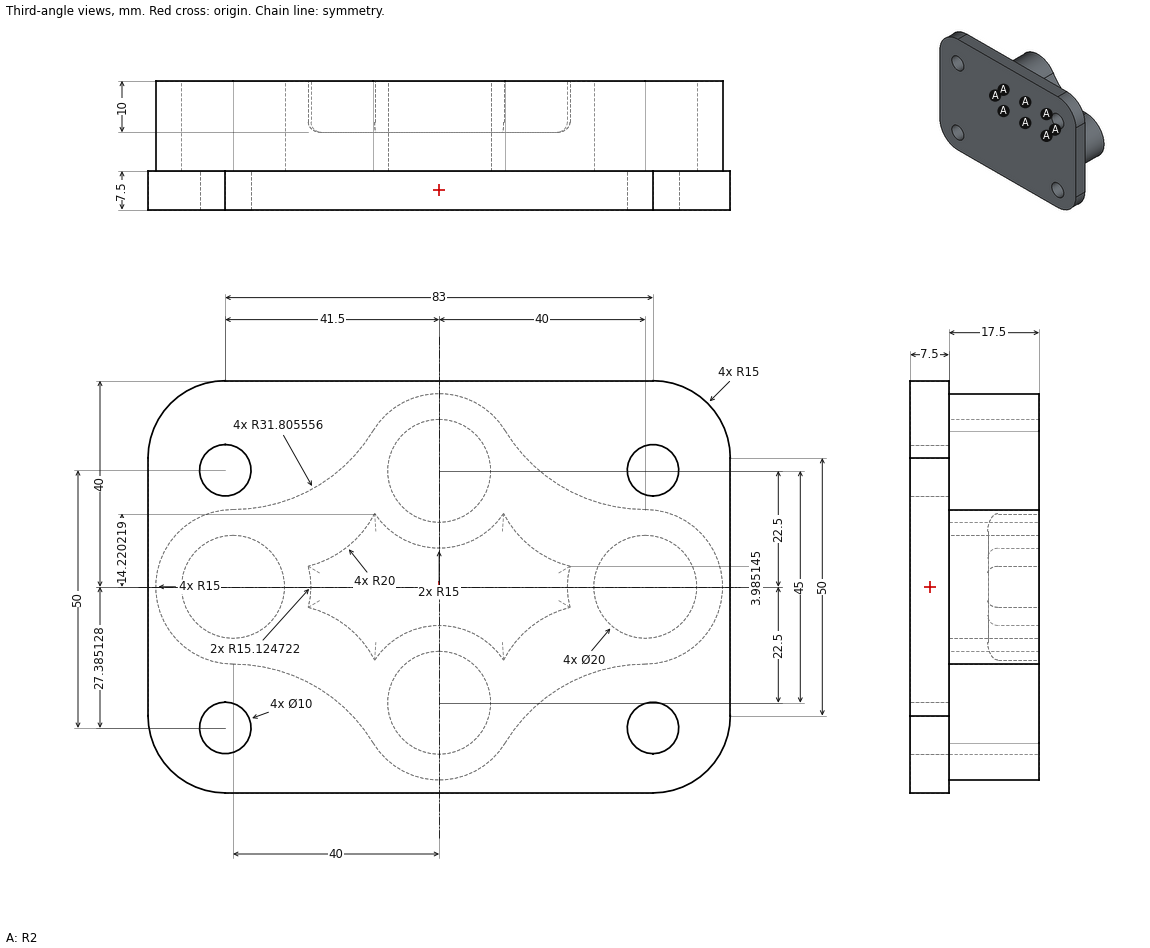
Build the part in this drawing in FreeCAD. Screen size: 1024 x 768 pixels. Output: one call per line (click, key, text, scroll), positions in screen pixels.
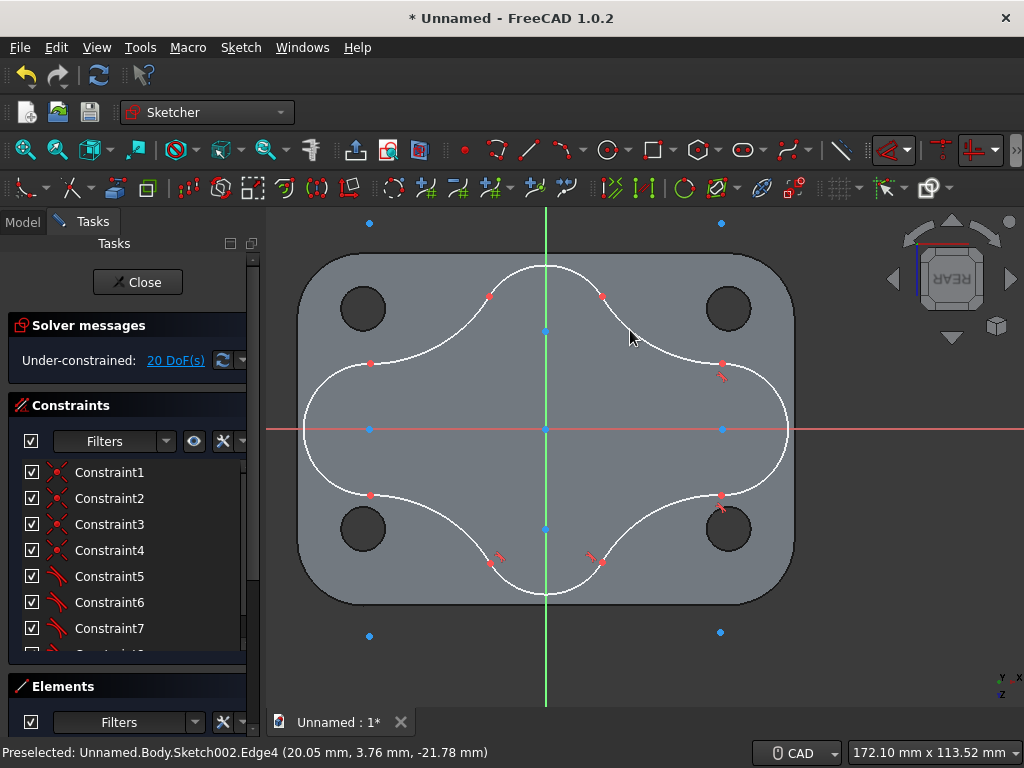
click(630, 330)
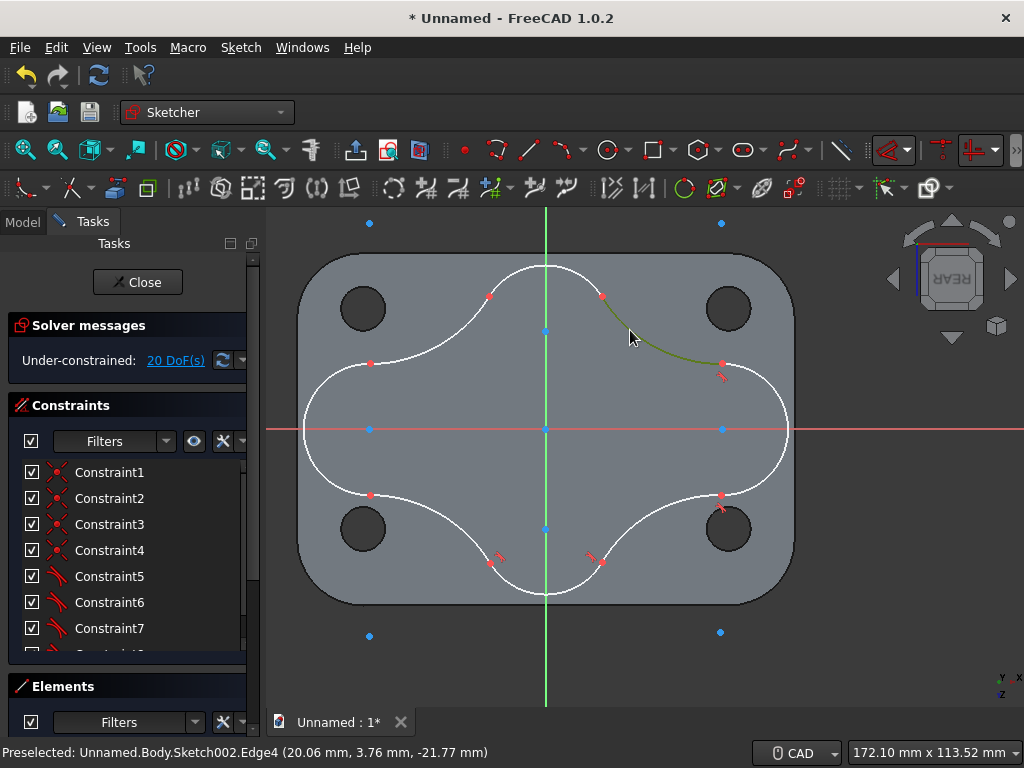
click(572, 271)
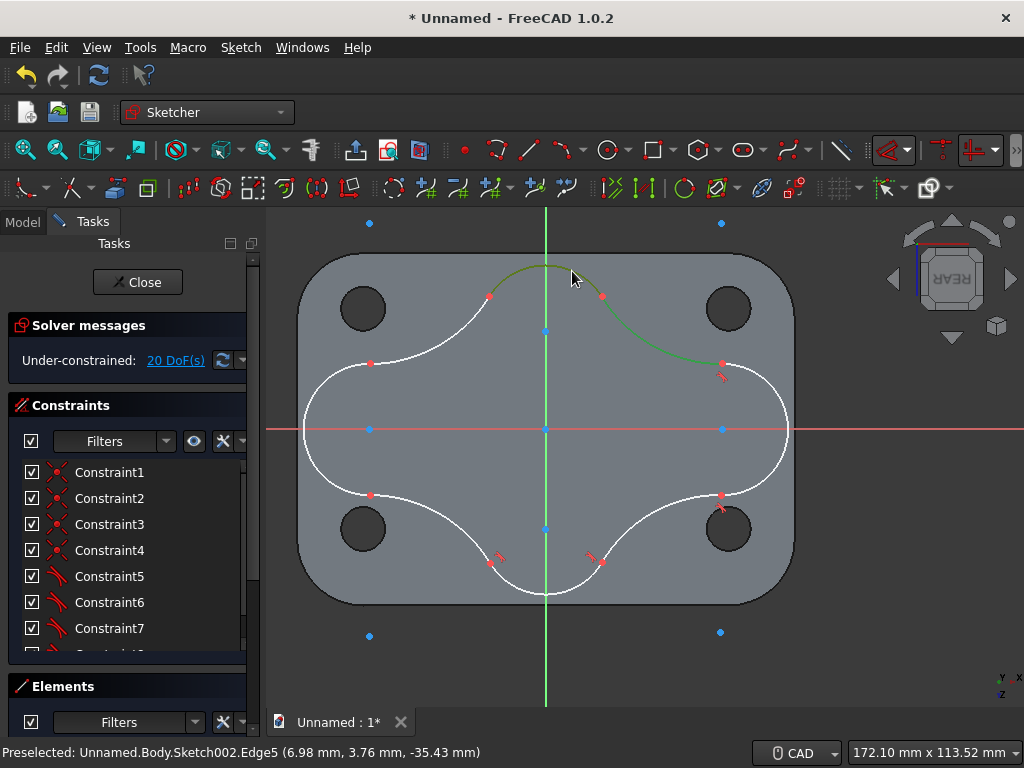
key(t)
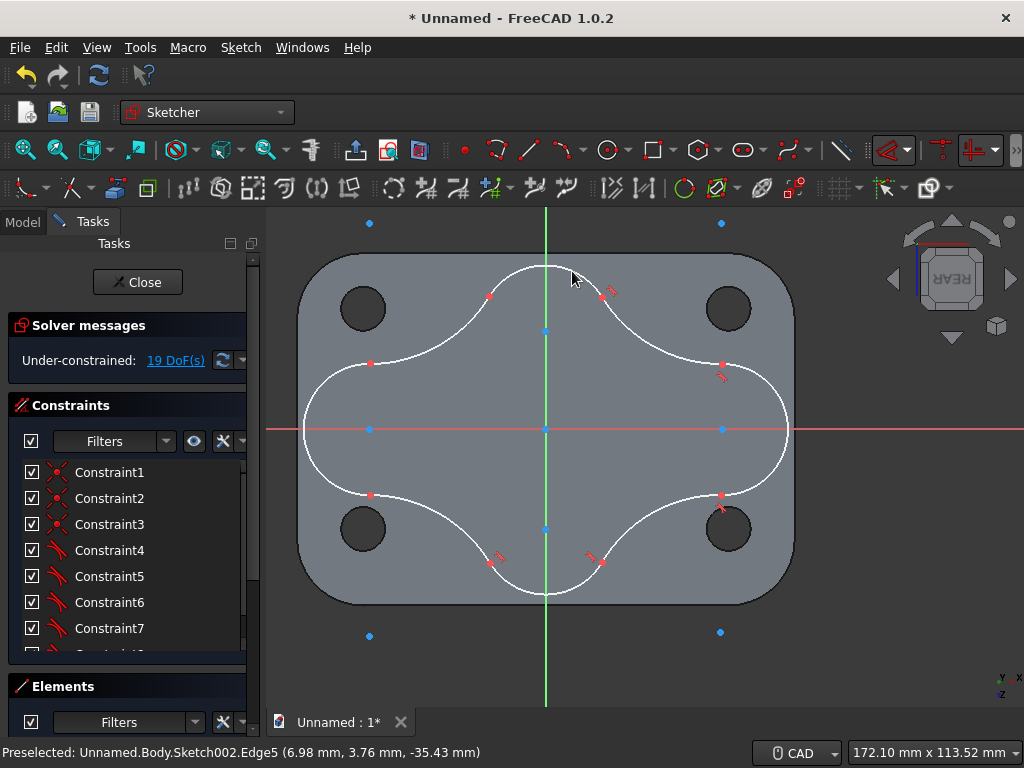
click(572, 271)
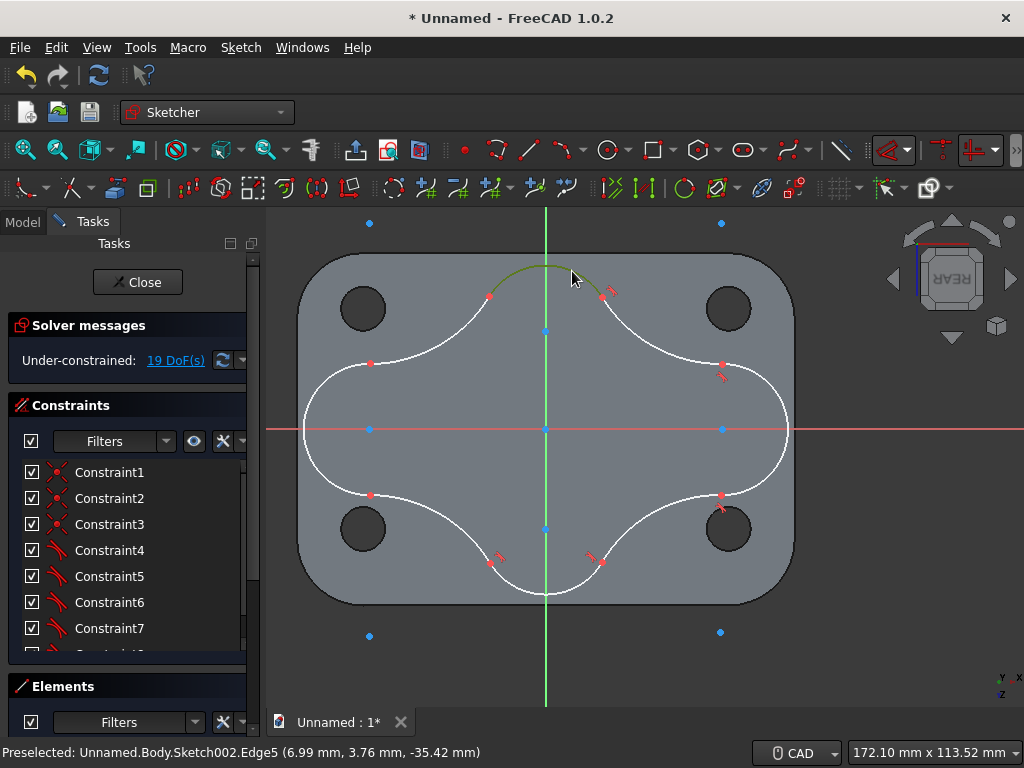
click(412, 357)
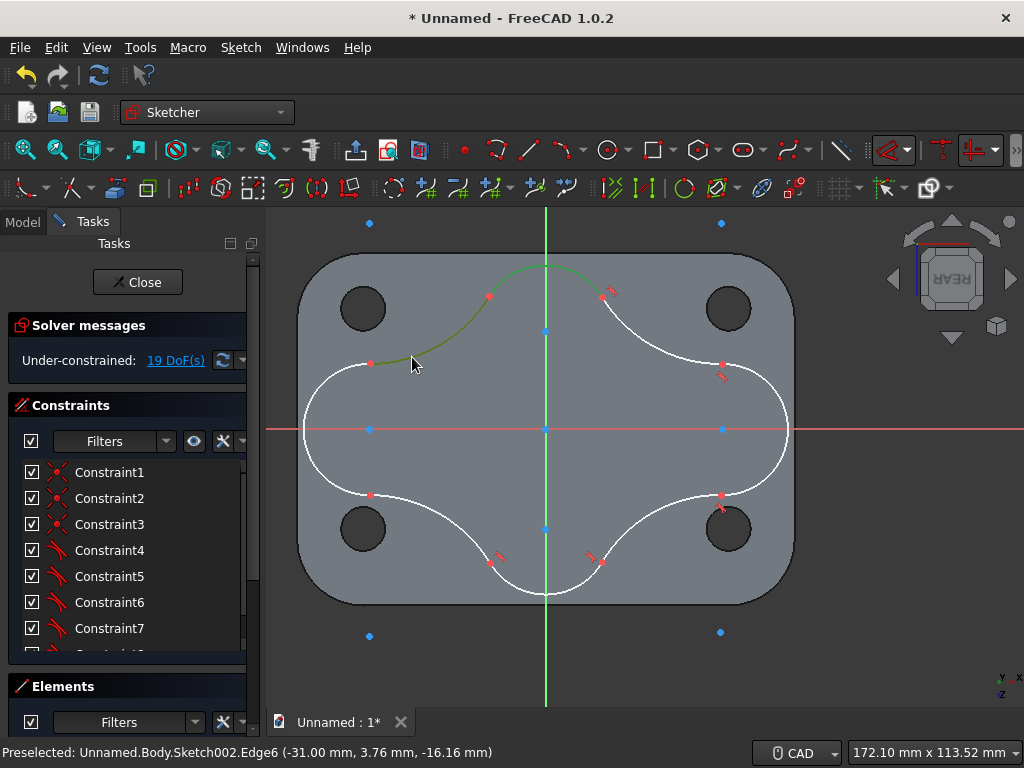
key(t)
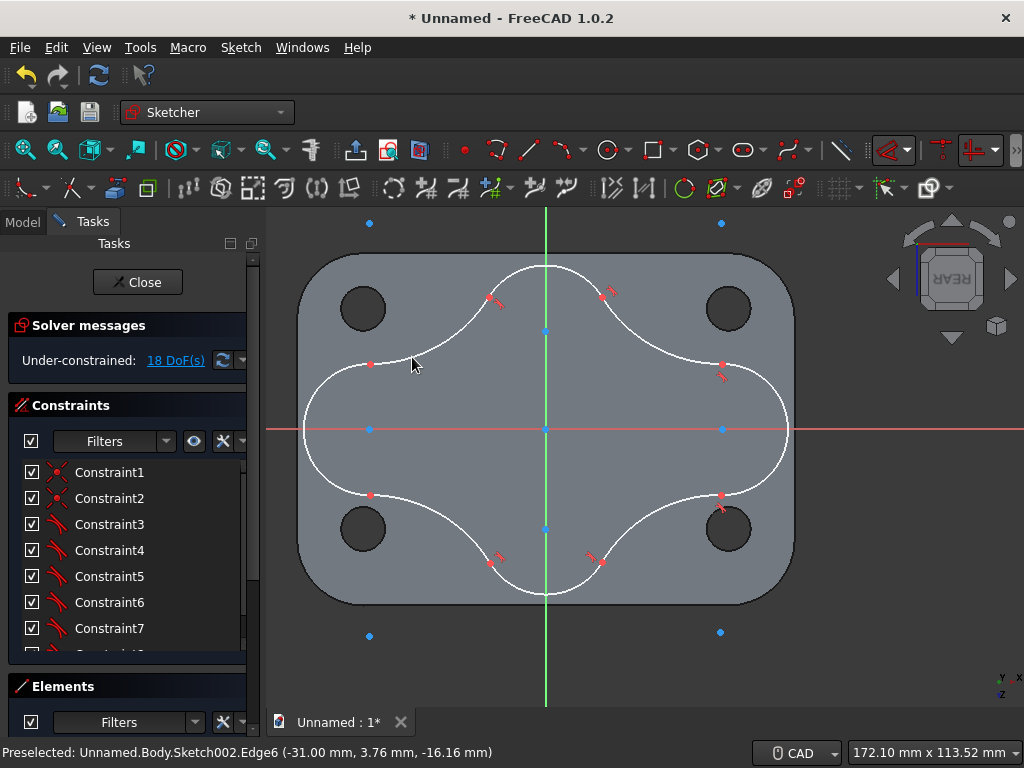
click(412, 357)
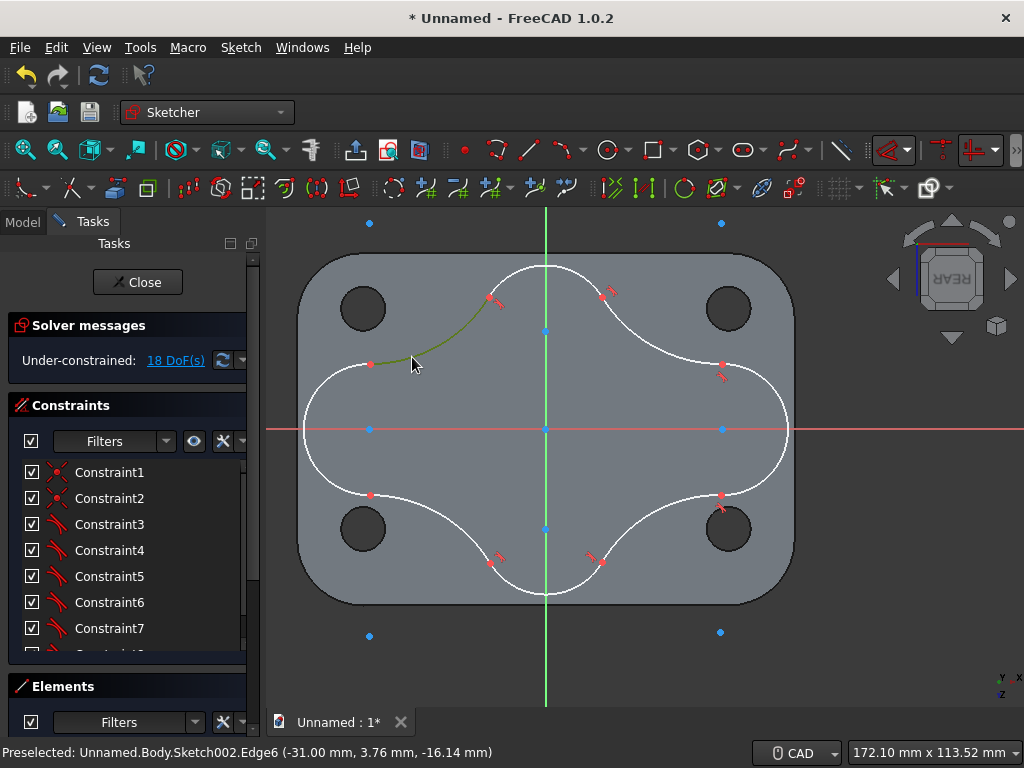
click(316, 391)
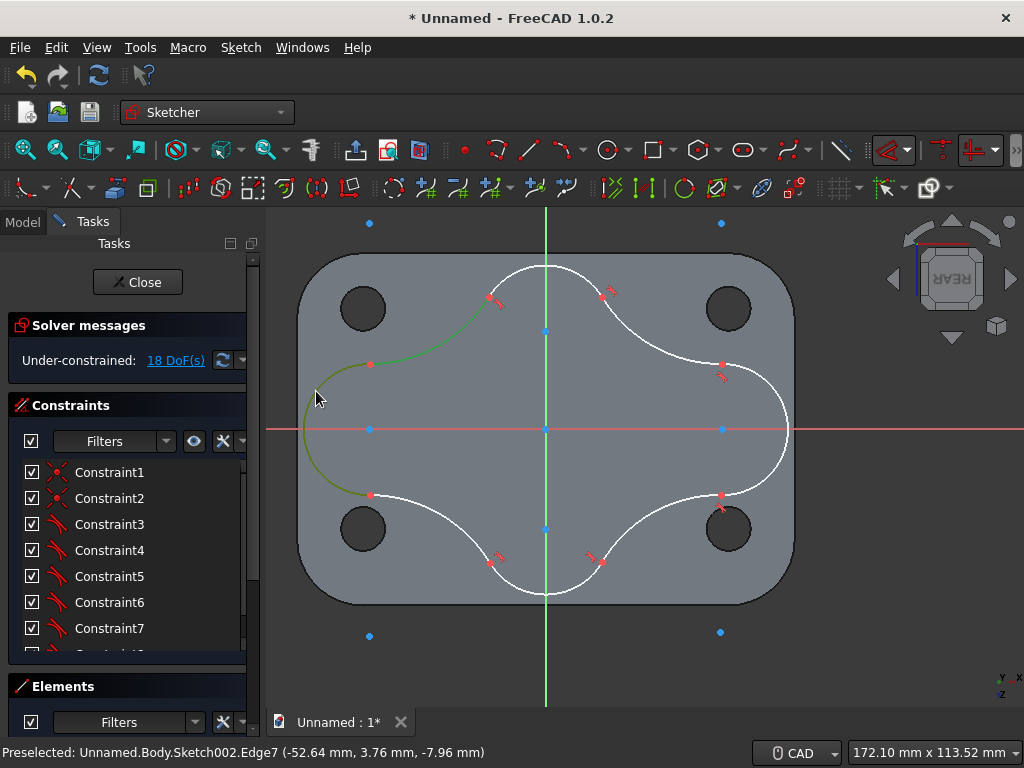
key(t)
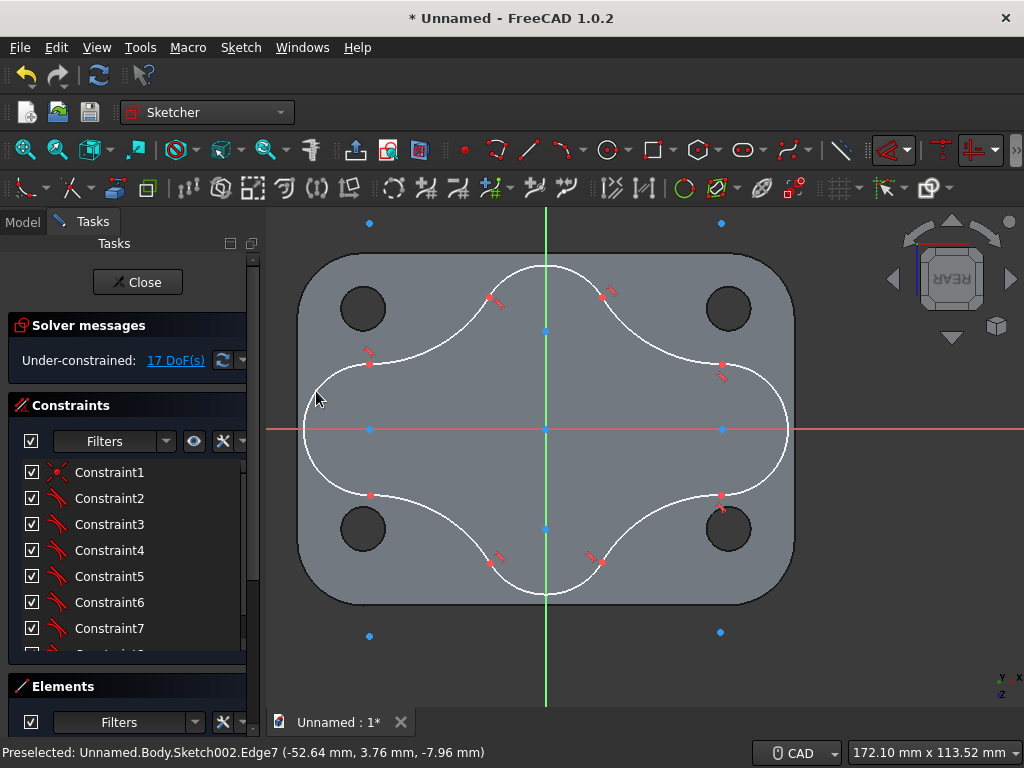
click(316, 391)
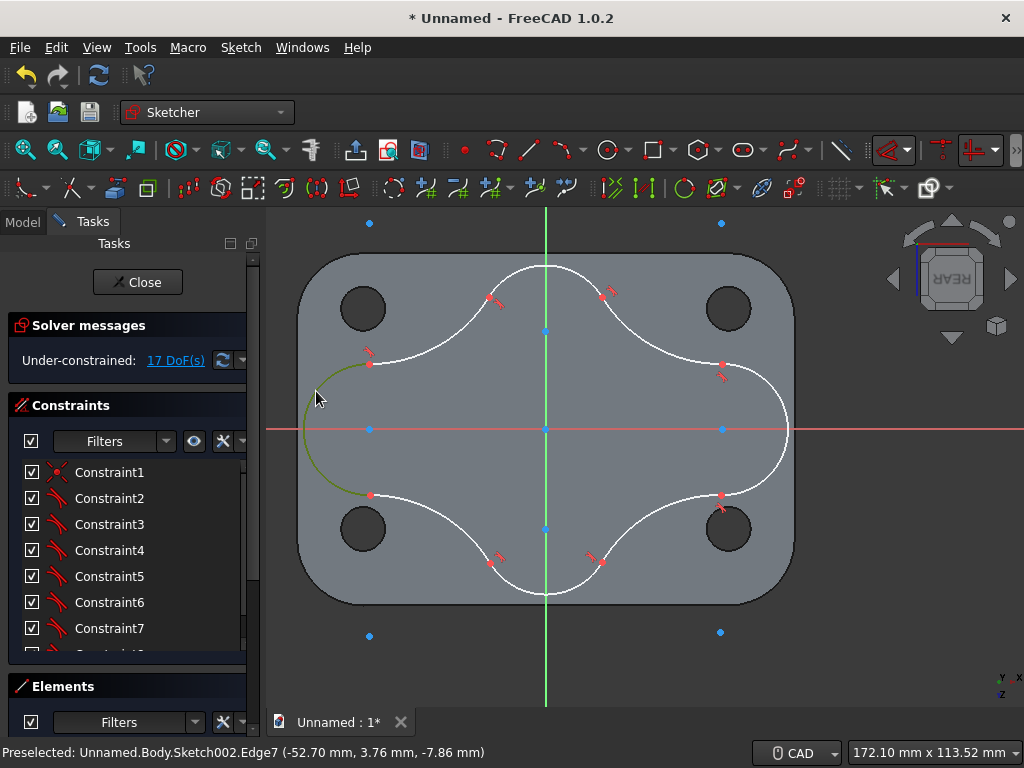
click(462, 530)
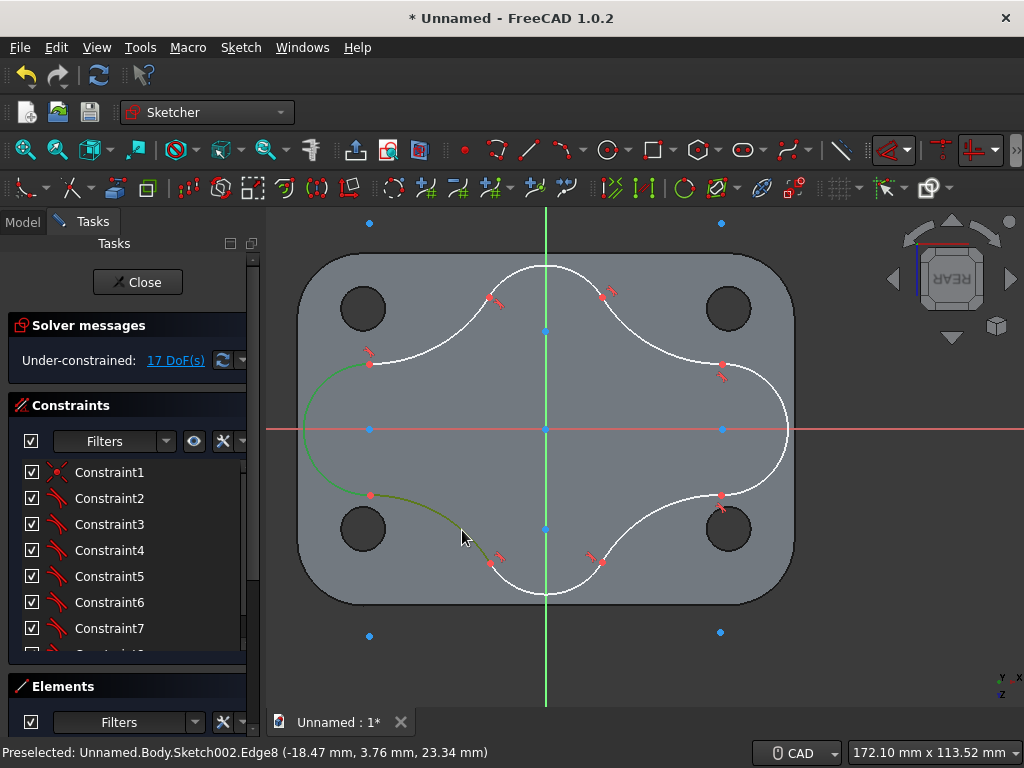
key(t)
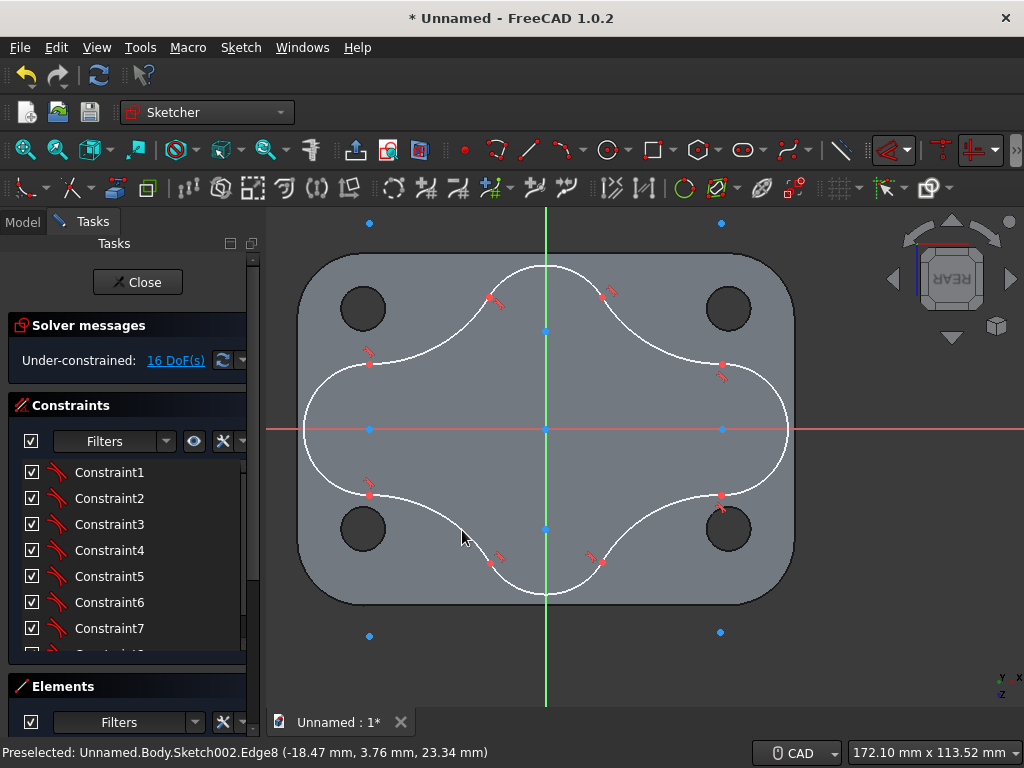
click(520, 589)